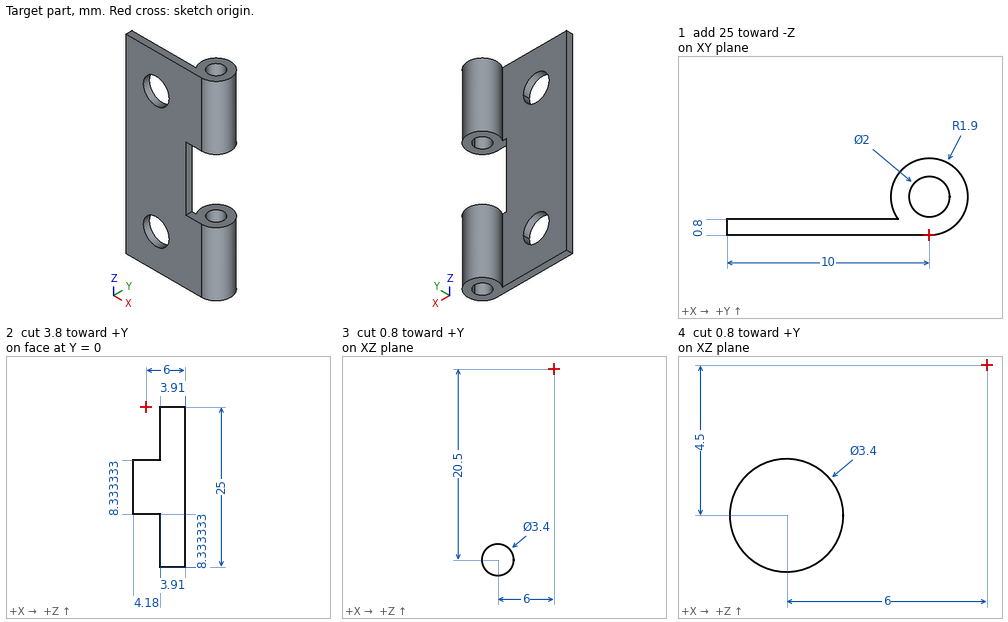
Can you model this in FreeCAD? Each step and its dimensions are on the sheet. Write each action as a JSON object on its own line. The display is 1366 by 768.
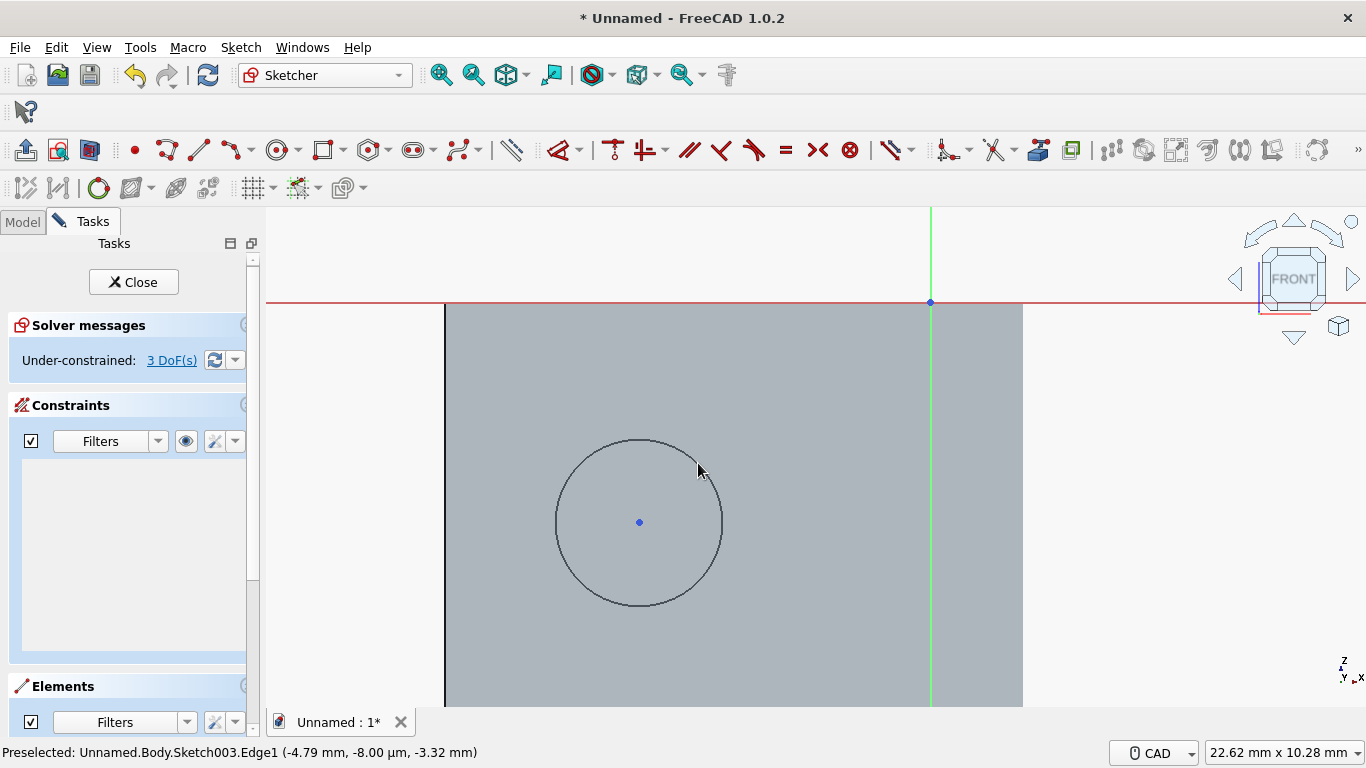
{"action": "left_click", "coordinate": [558, 150]}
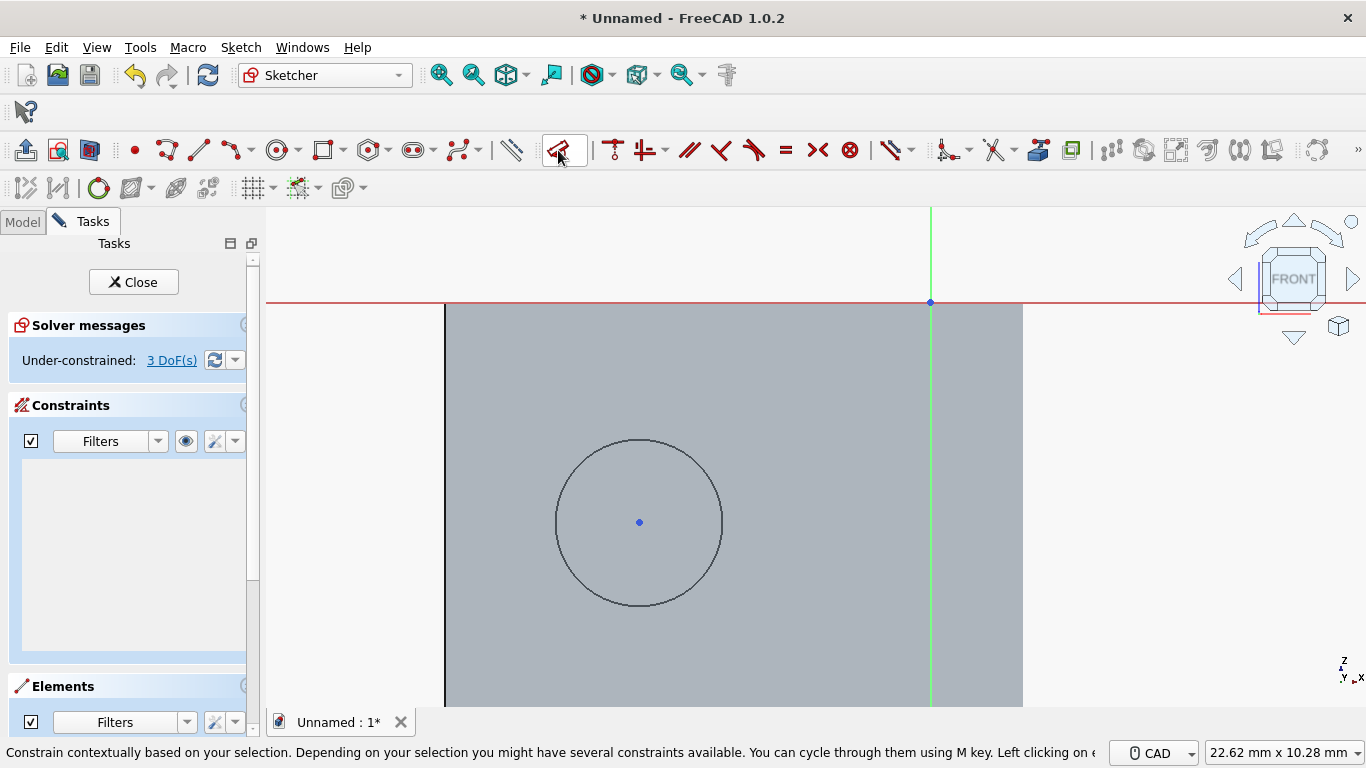
{"action": "left_click", "coordinate": [698, 464]}
{"action": "left_click", "coordinate": [721, 441]}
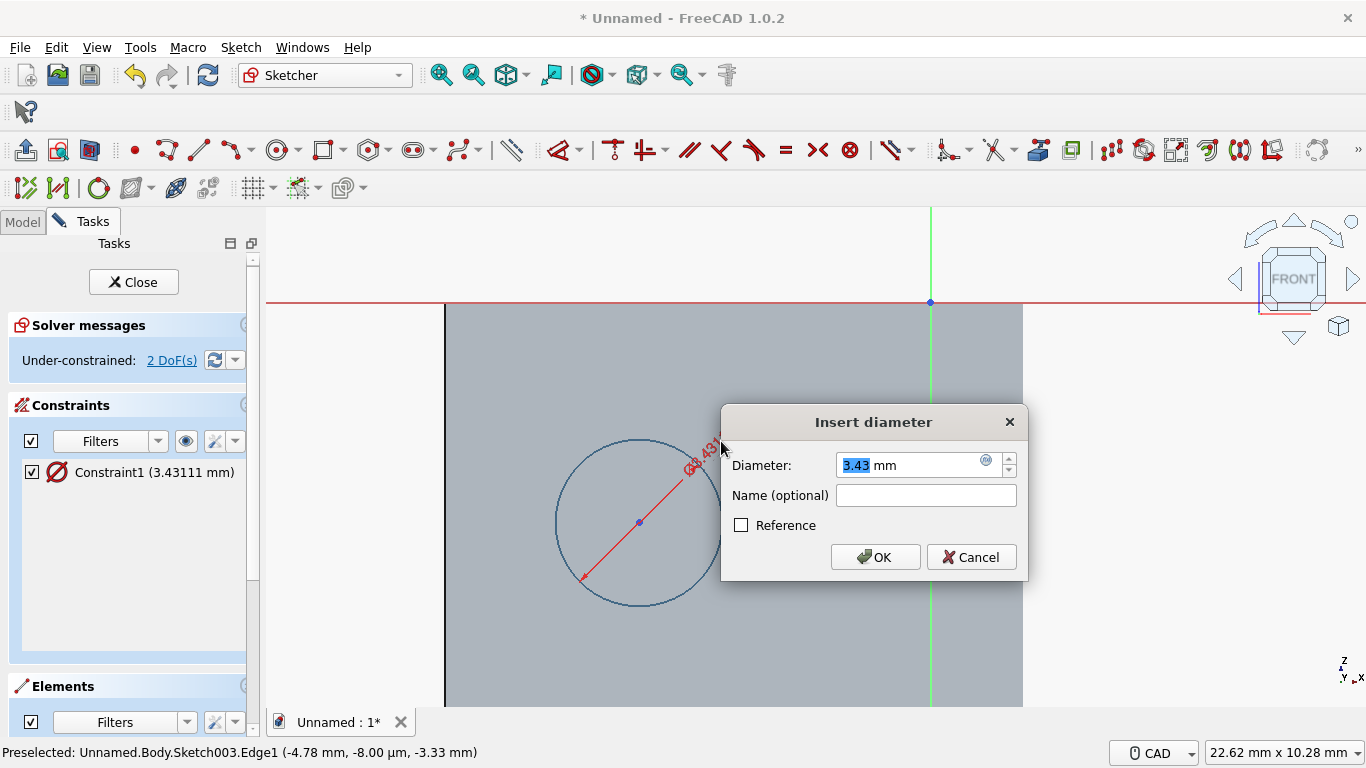
{"action": "type", "text": "3.4"}
{"action": "key", "text": "Return"}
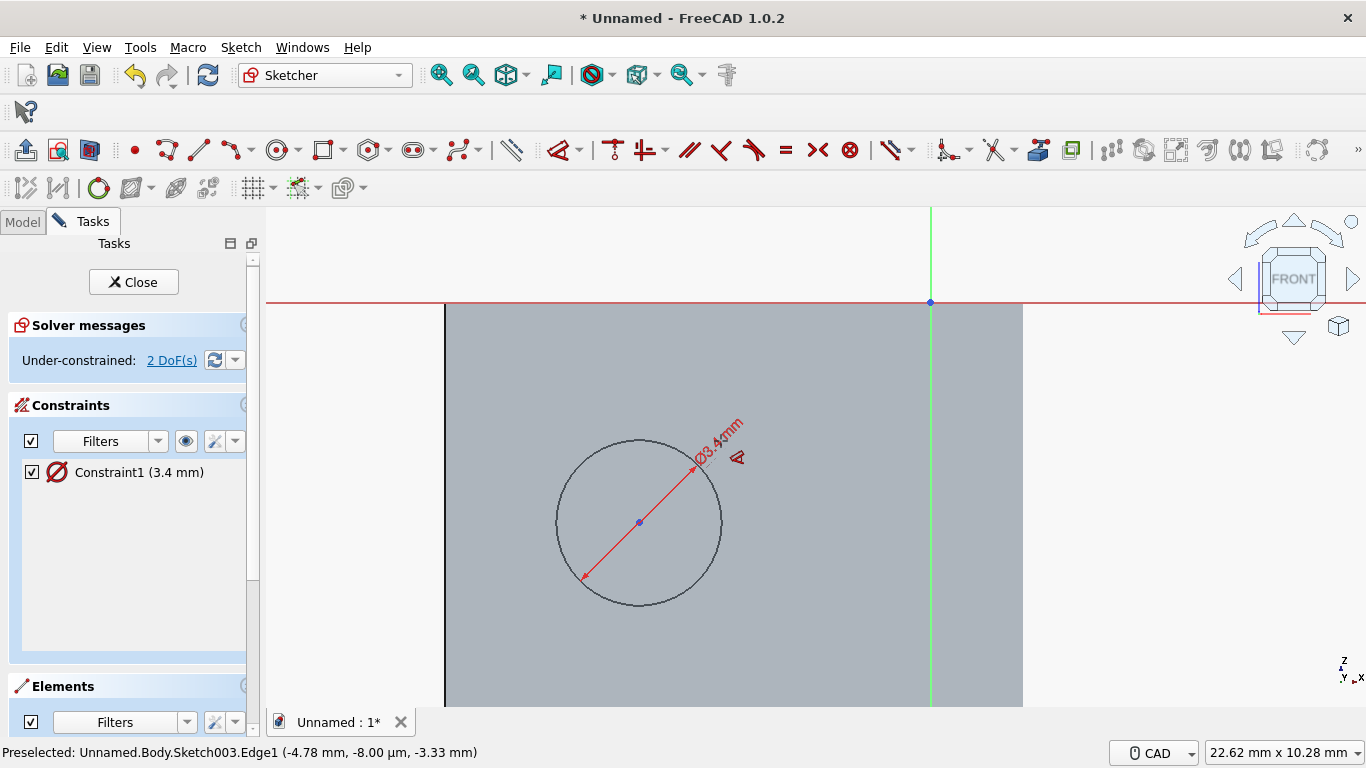
{"action": "left_click", "coordinate": [639, 523]}
{"action": "left_click", "coordinate": [785, 269]}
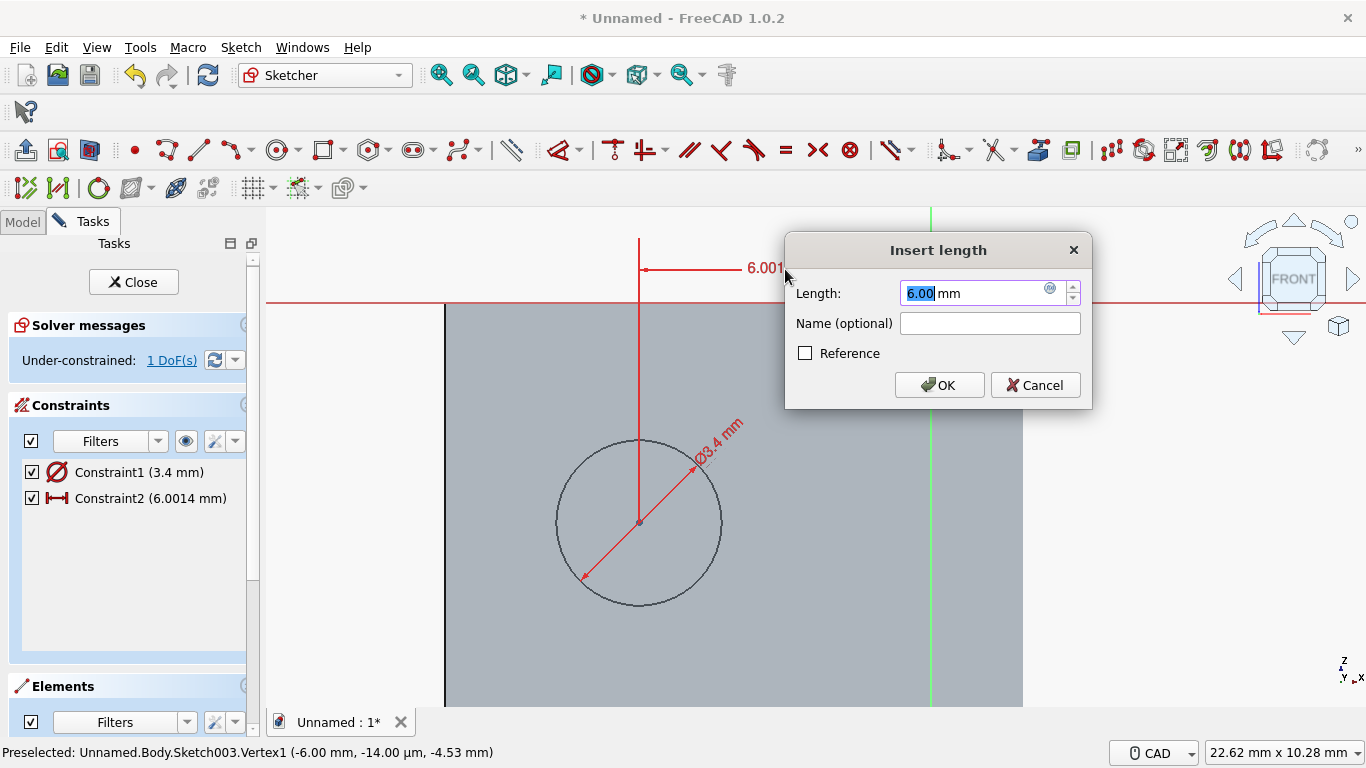
{"action": "type", "text": "6"}
{"action": "key", "text": "Return"}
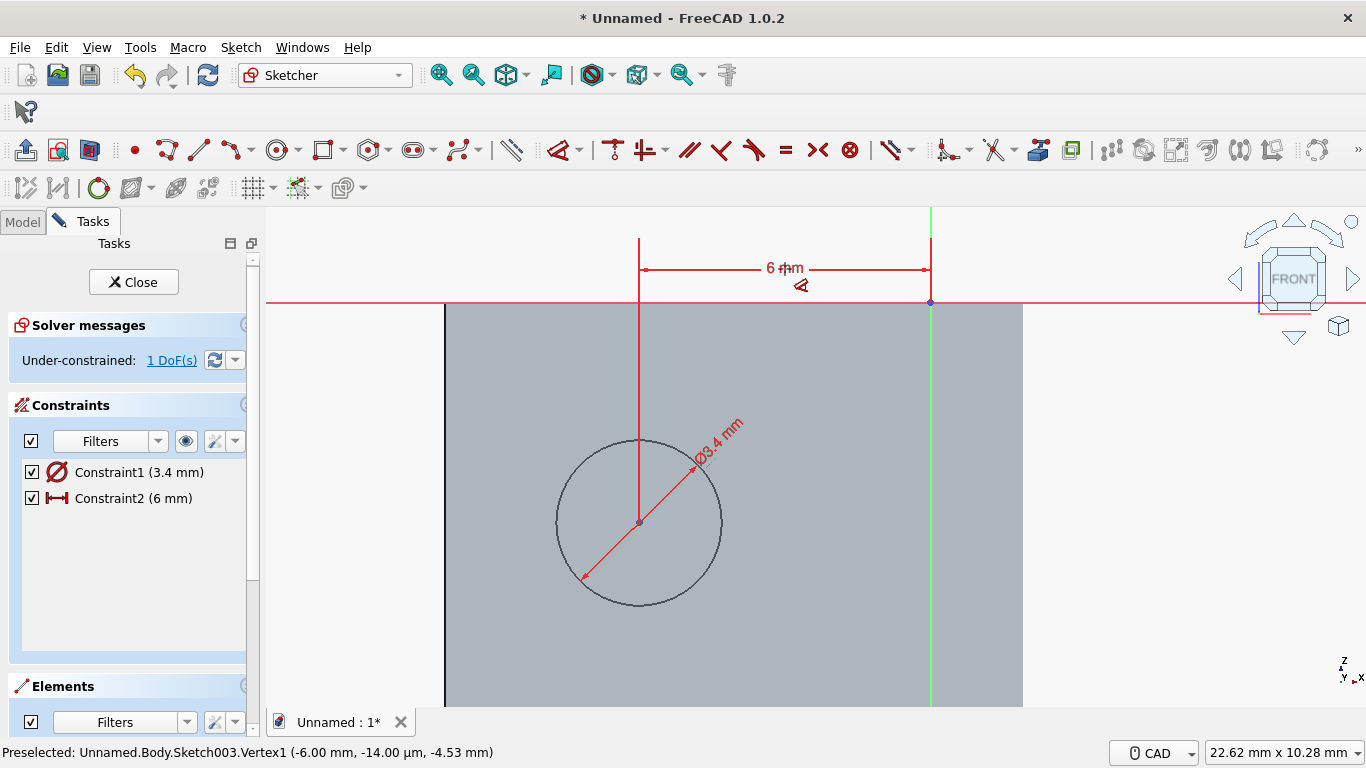
{"action": "left_click", "coordinate": [639, 523]}
{"action": "left_click", "coordinate": [965, 413]}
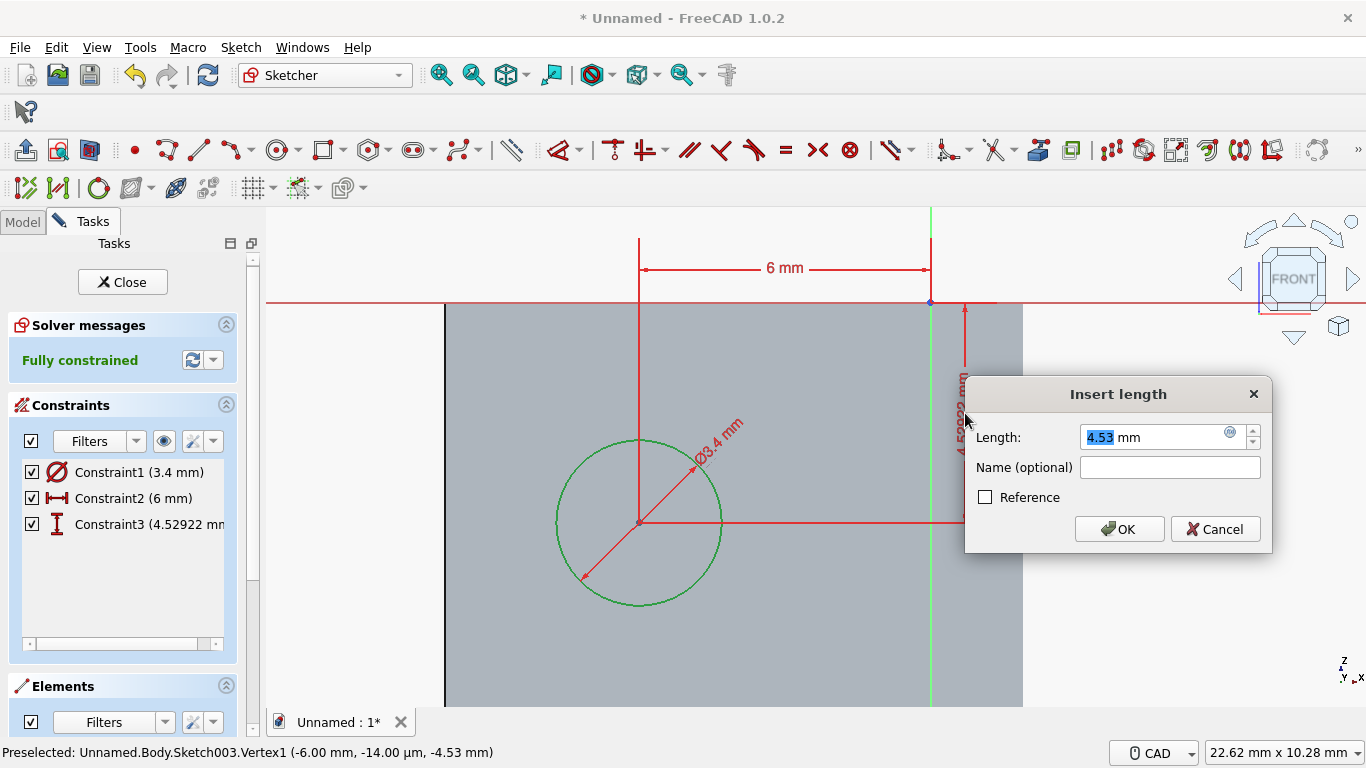
{"action": "type", "text": "4.5"}
{"action": "key", "text": "Return"}
{"action": "key", "text": "Escape"}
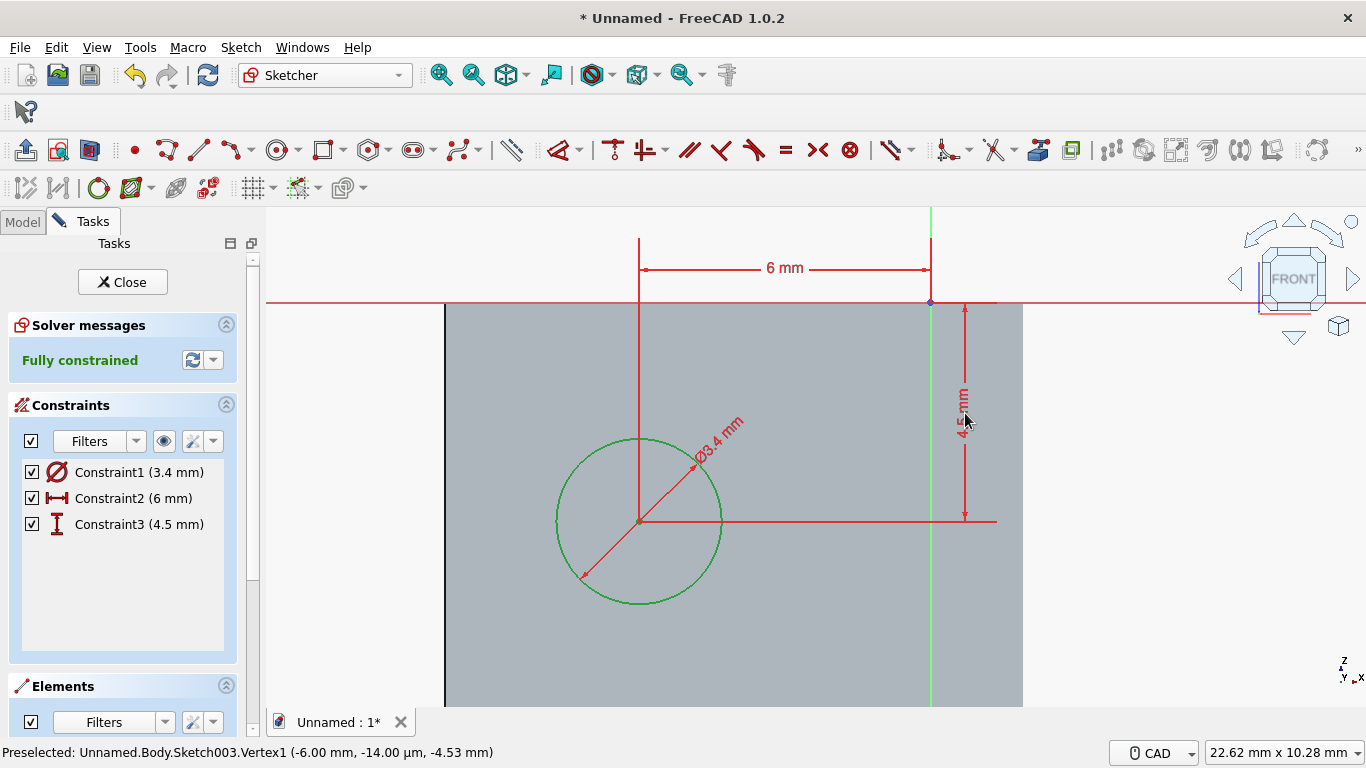
{"action": "left_click", "coordinate": [123, 282]}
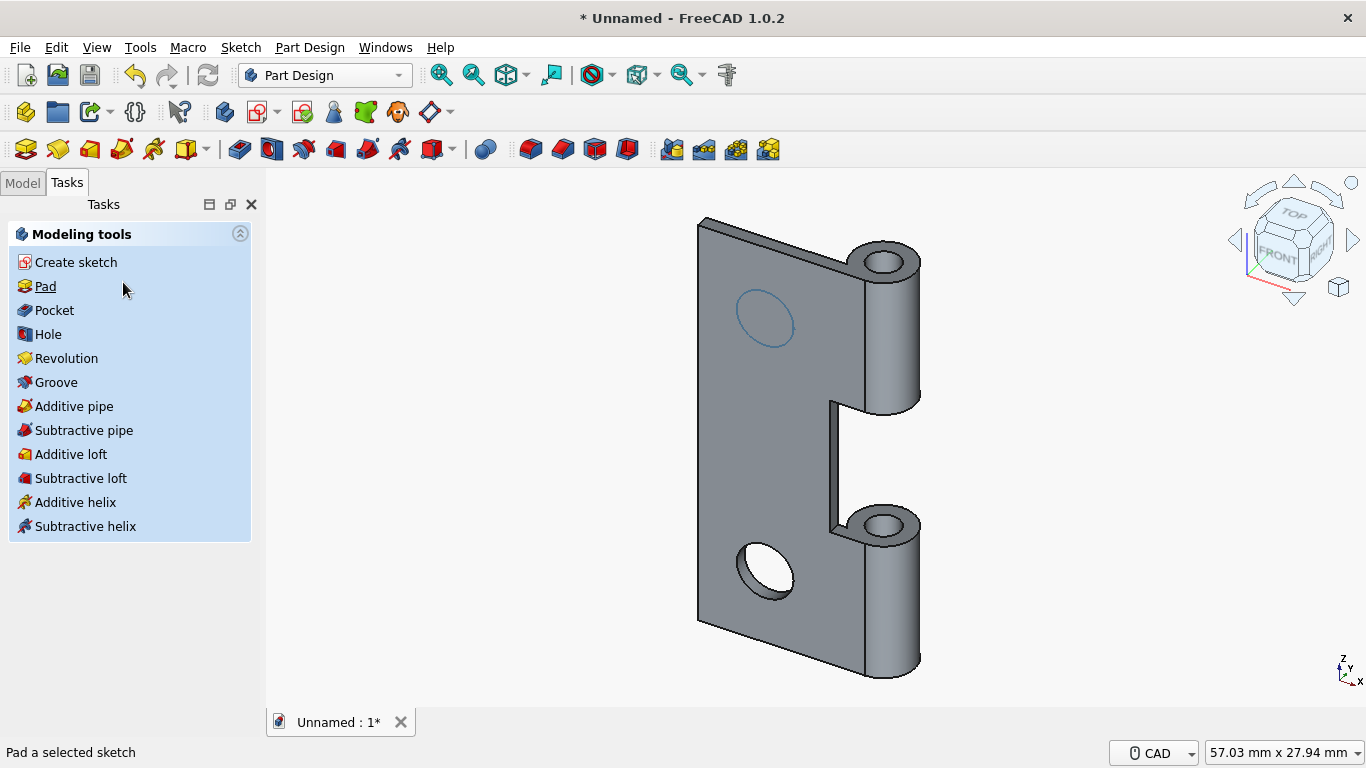
{"action": "left_click", "coordinate": [240, 150]}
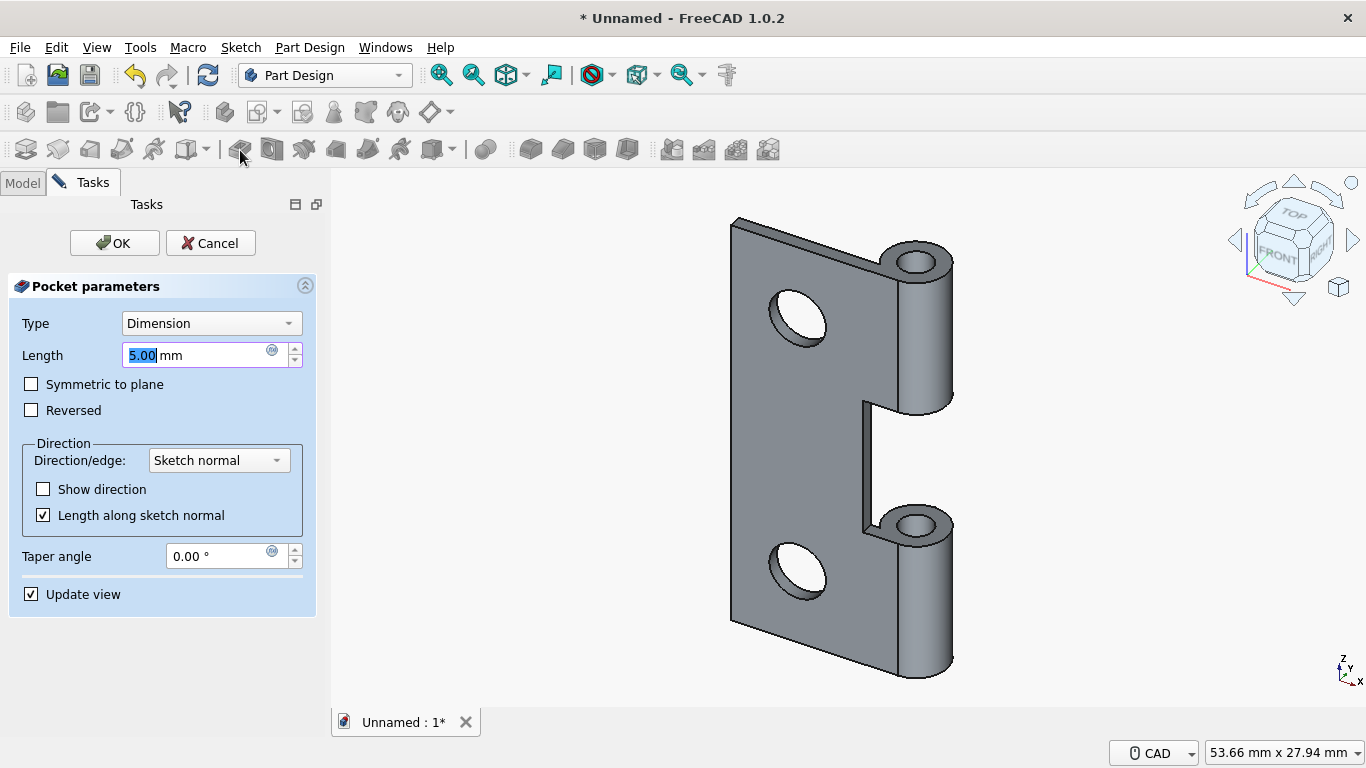
{"action": "type", "text": "0.8"}
{"action": "key", "text": "Tab"}